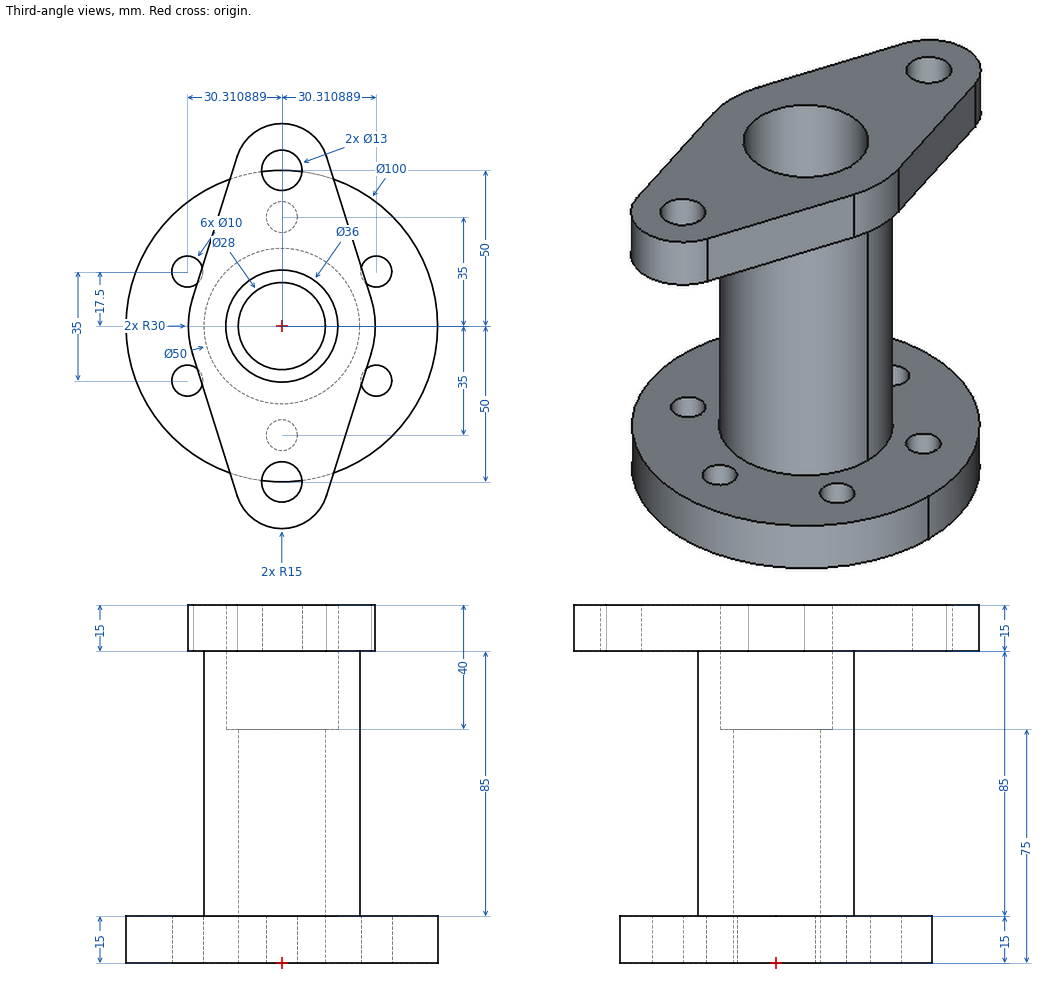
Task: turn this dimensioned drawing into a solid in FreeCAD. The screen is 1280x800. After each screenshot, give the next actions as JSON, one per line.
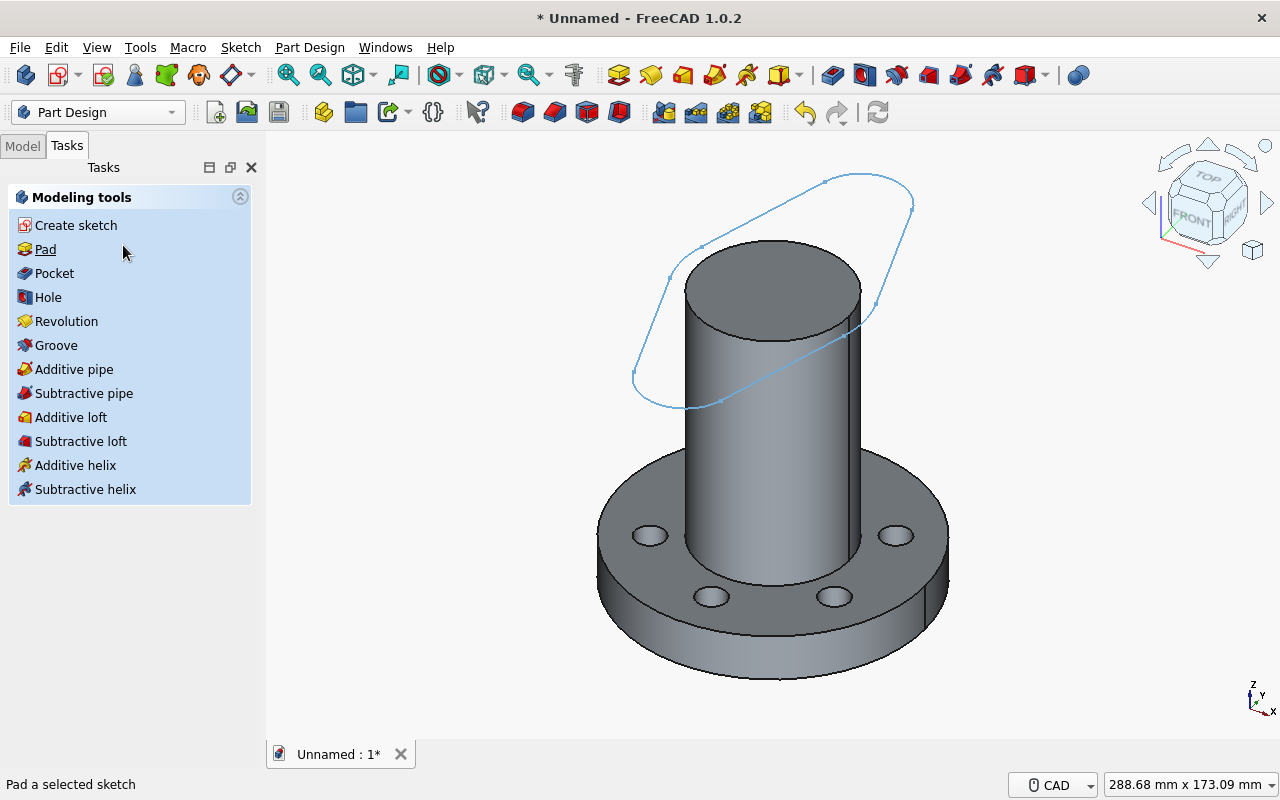
{"action": "left_click", "coordinate": [620, 76]}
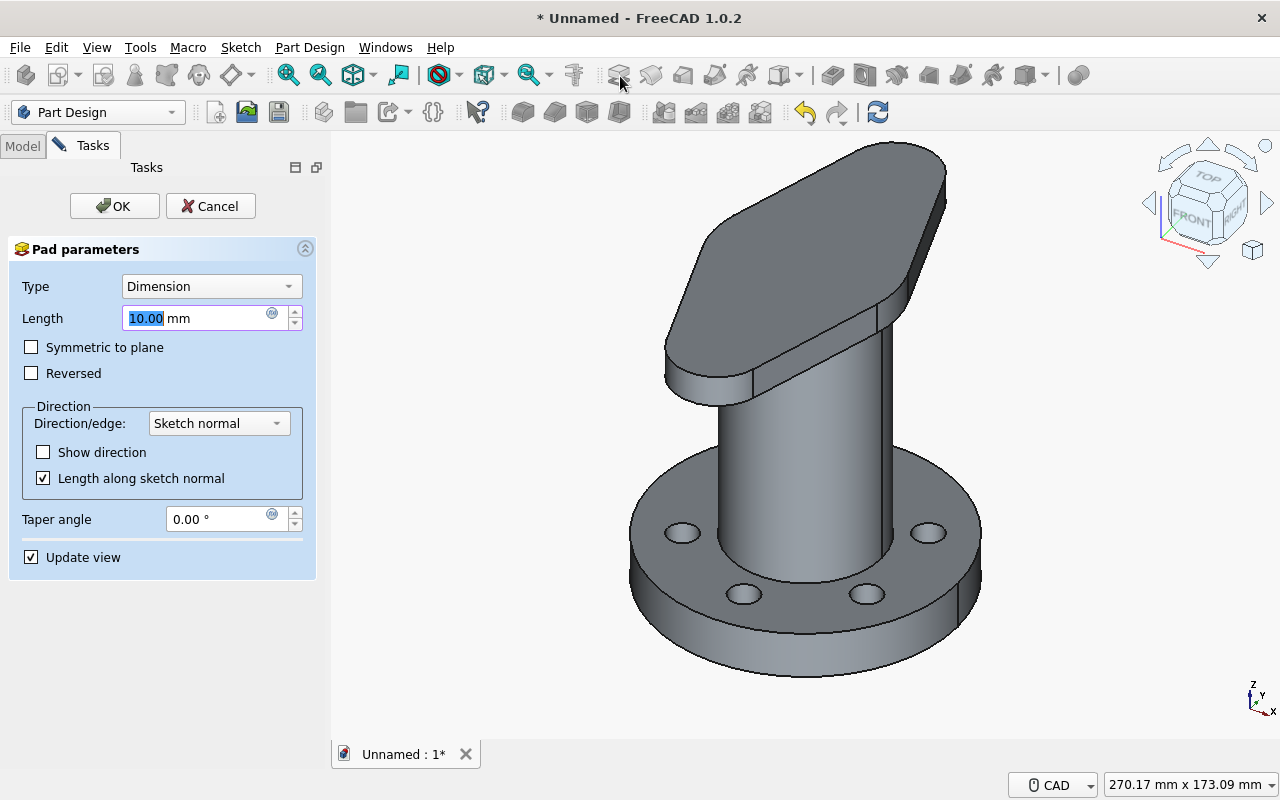
{"action": "type", "text": "15"}
{"action": "key", "text": "Tab"}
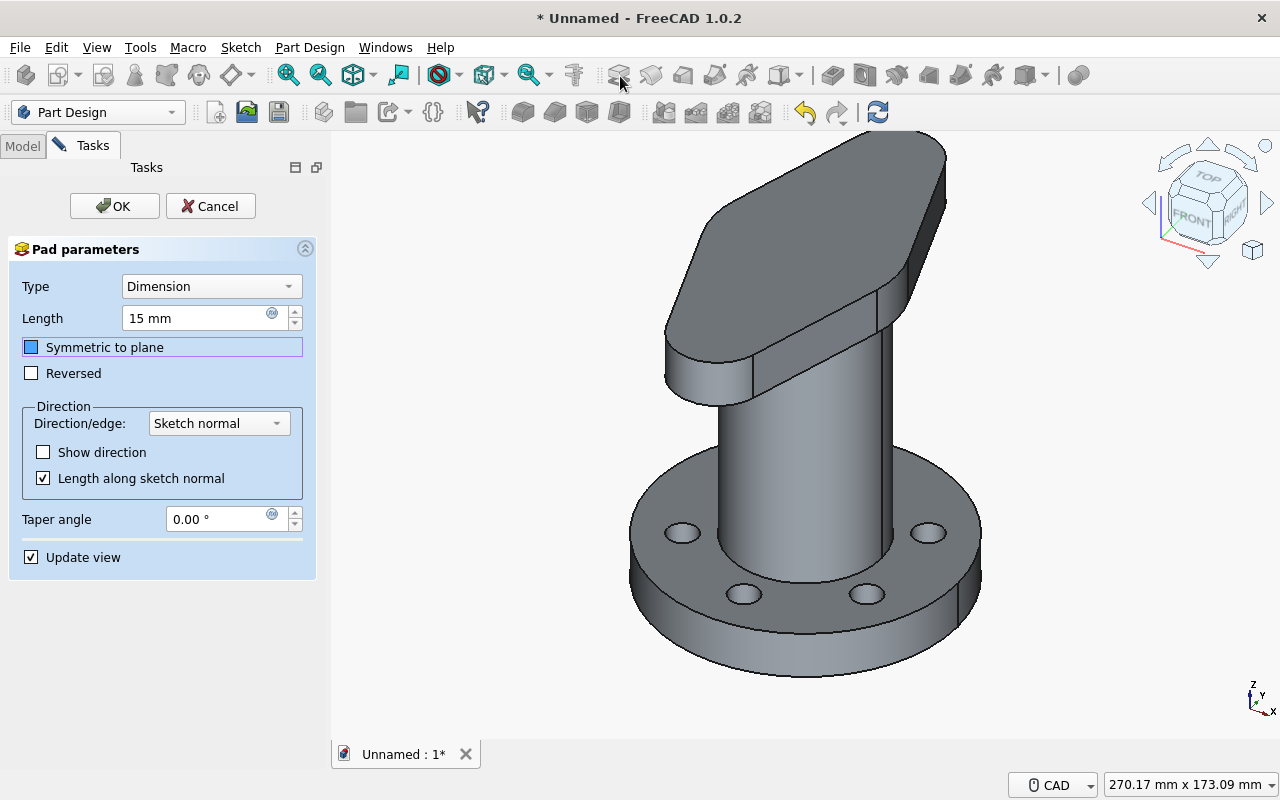
{"action": "left_click", "coordinate": [115, 206]}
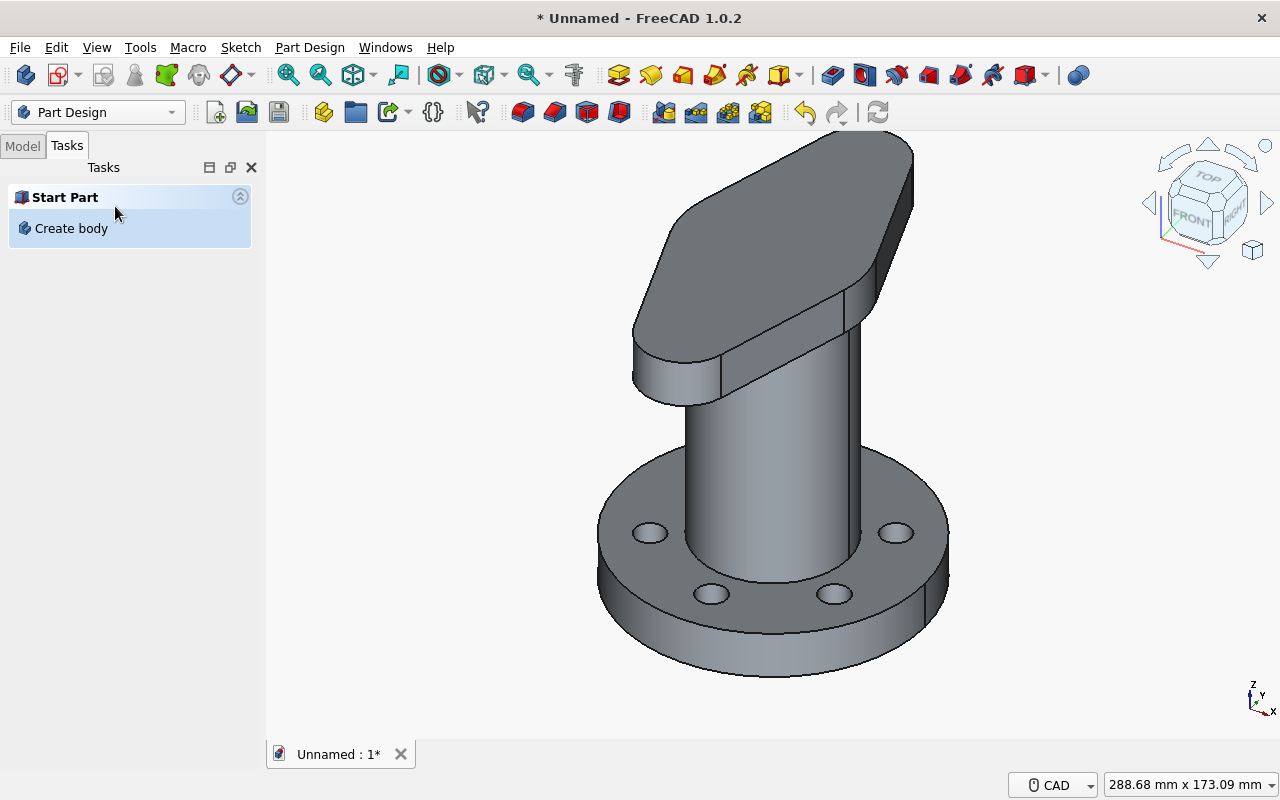
{"action": "key", "text": "v f"}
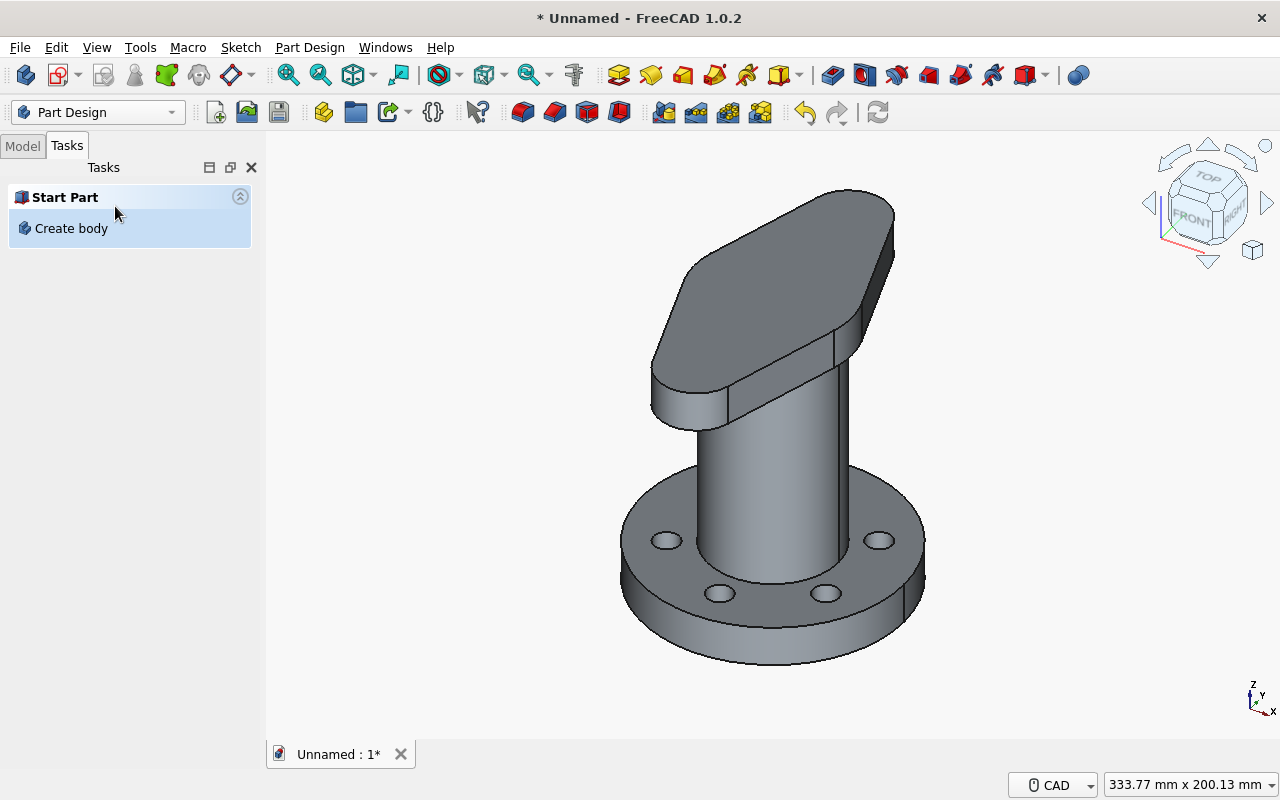
{"action": "left_click", "coordinate": [773, 291]}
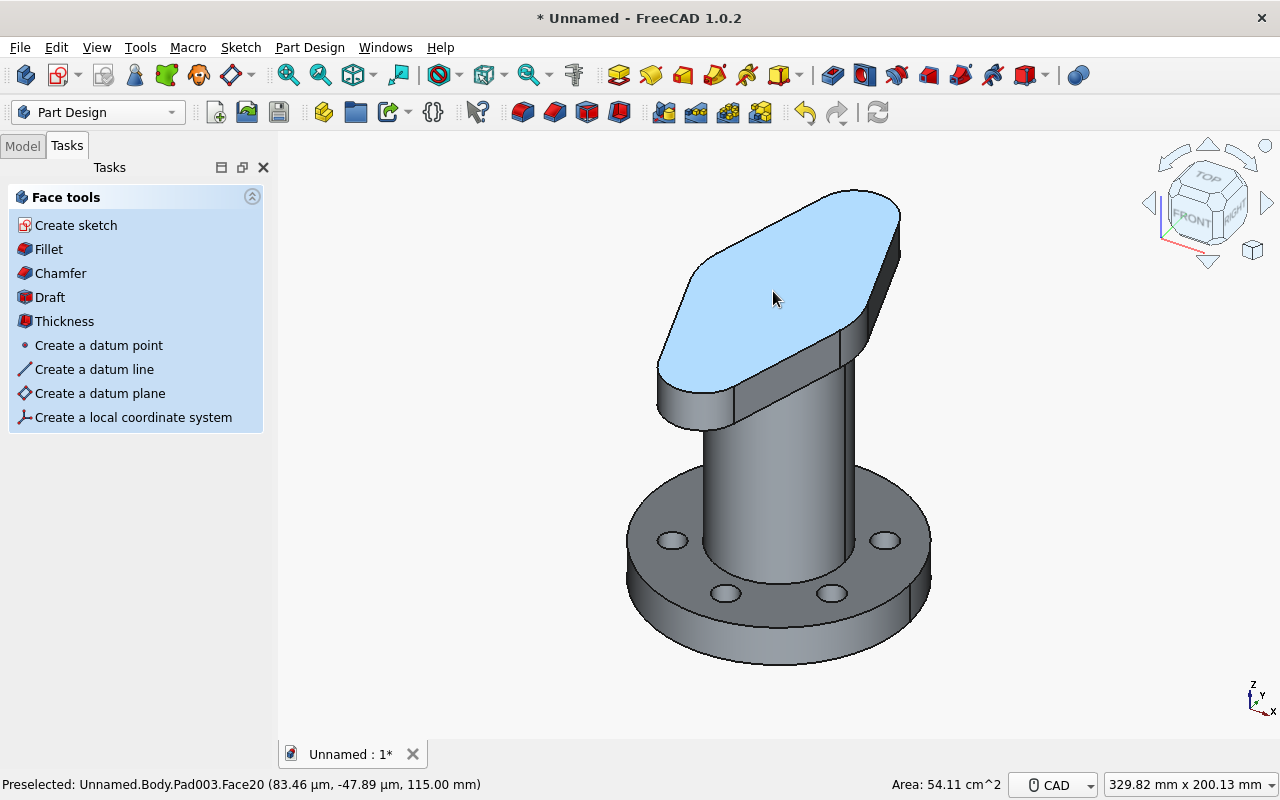
{"action": "left_click", "coordinate": [58, 76]}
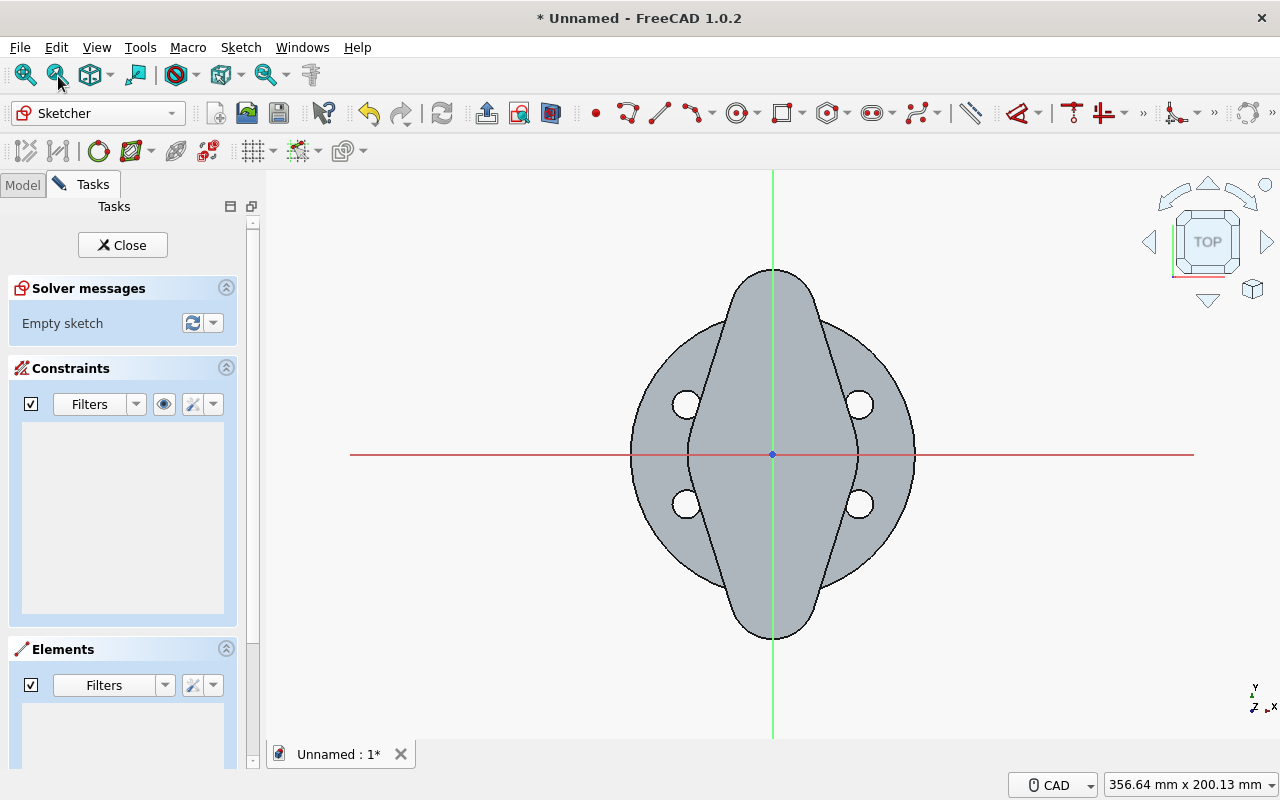
{"action": "key", "text": "g c"}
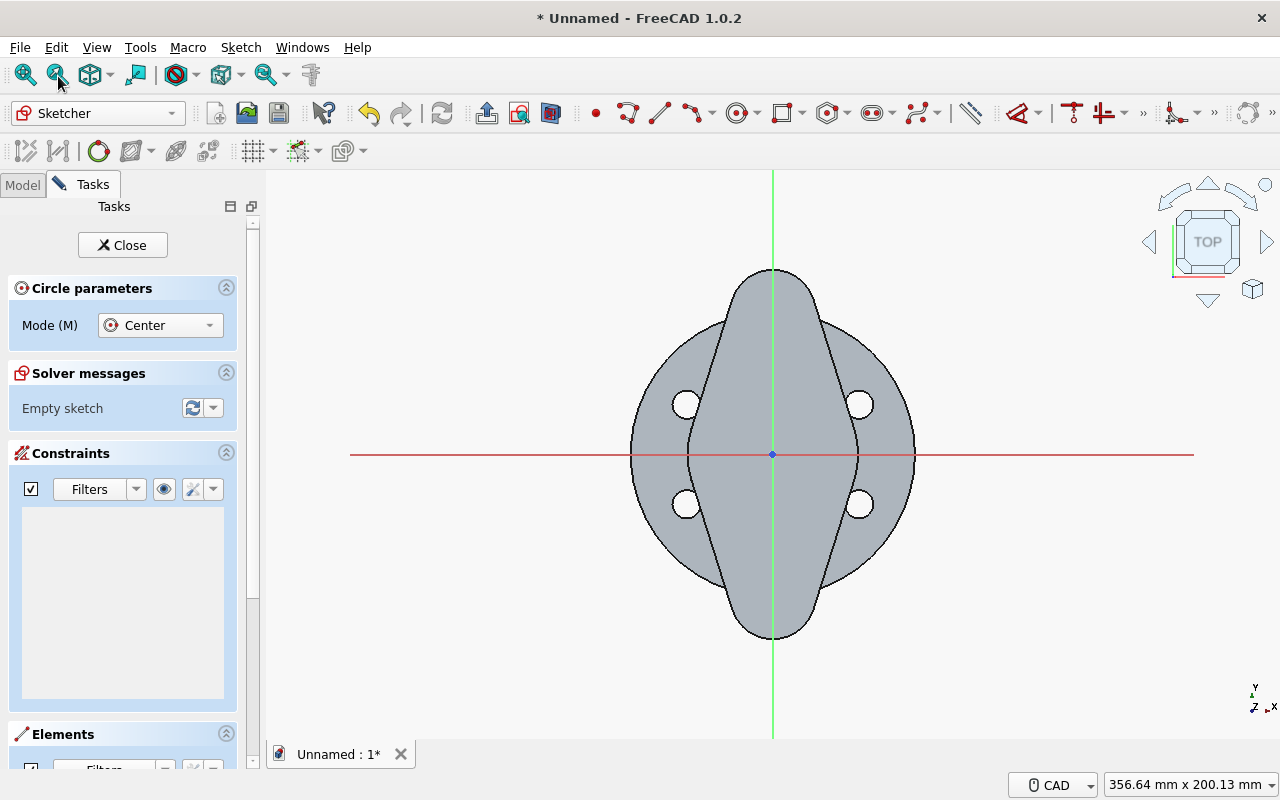
{"action": "scroll", "coordinate": [773, 312], "scroll_direction": "up", "scroll_amount": 2}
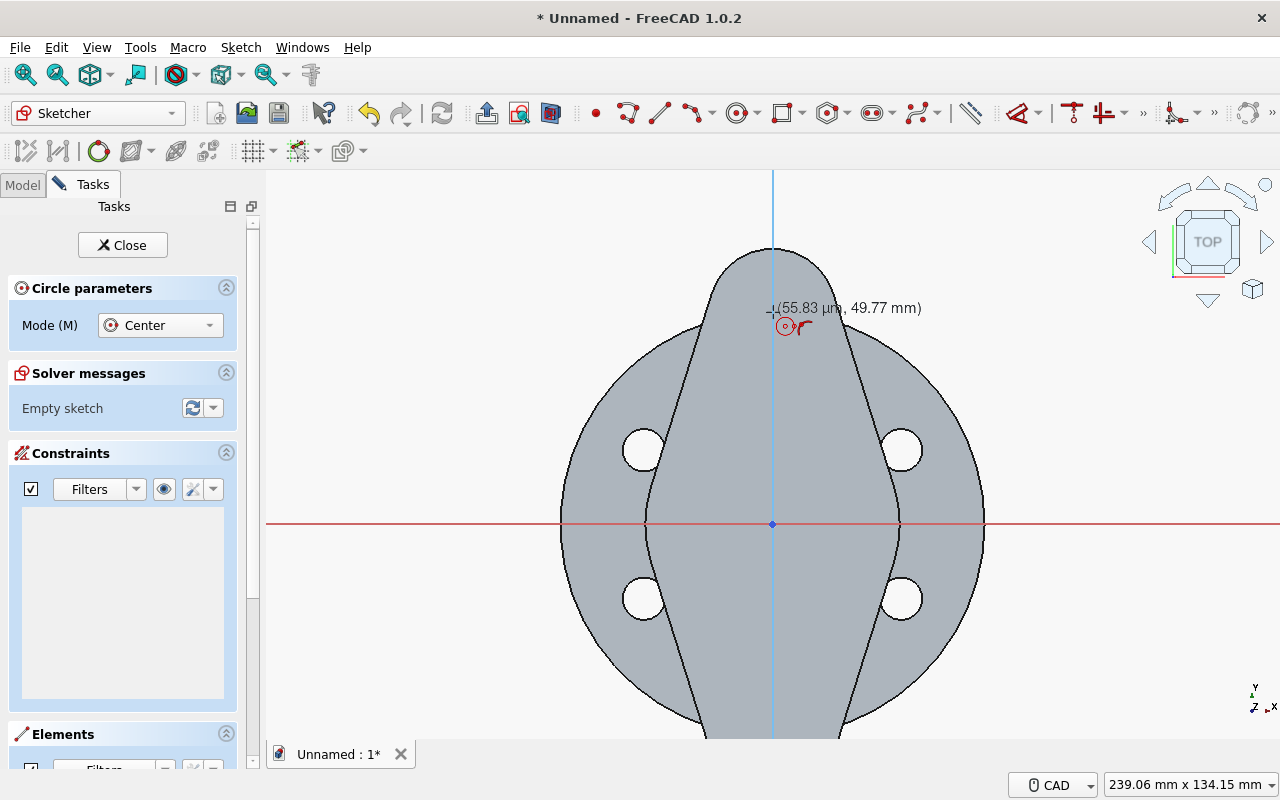
{"action": "left_click", "coordinate": [773, 312]}
{"action": "mouse_move", "coordinate": [792, 293]}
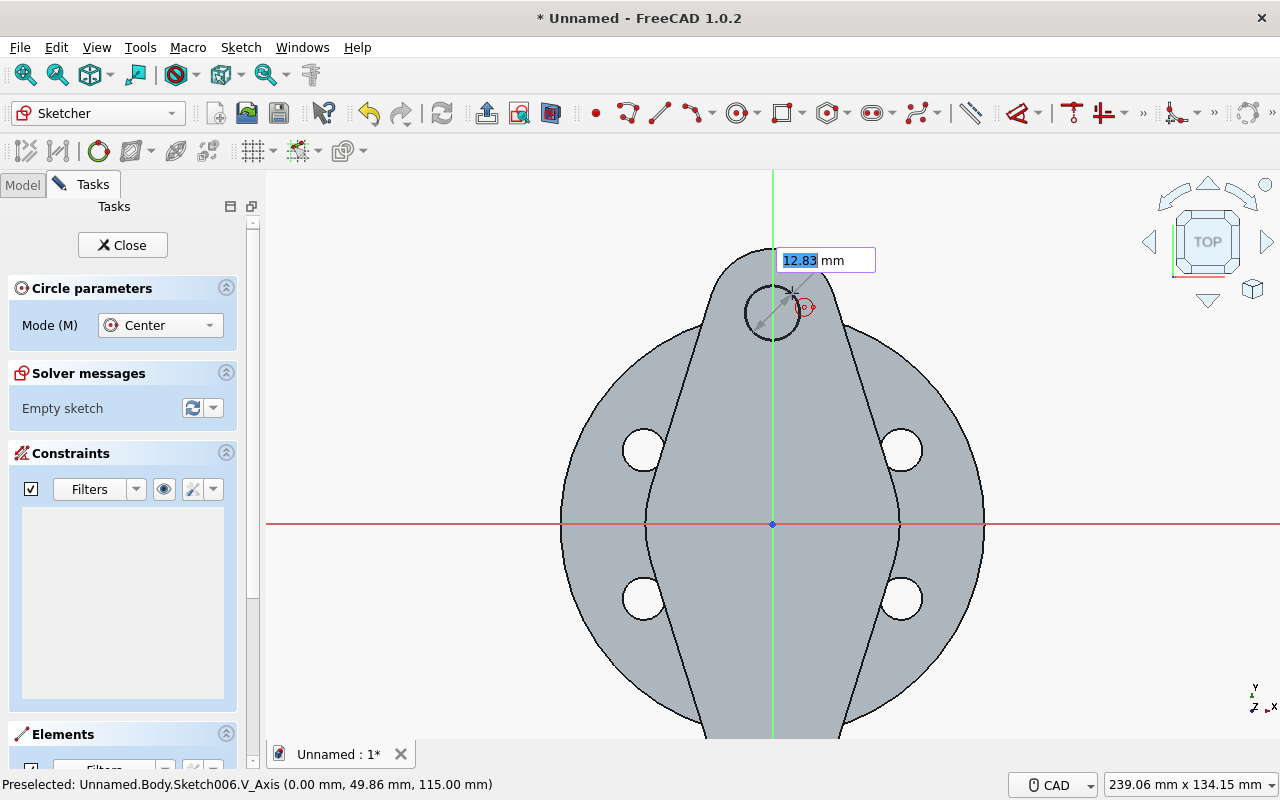
{"action": "type", "text": "13"}
{"action": "key", "text": "Return"}